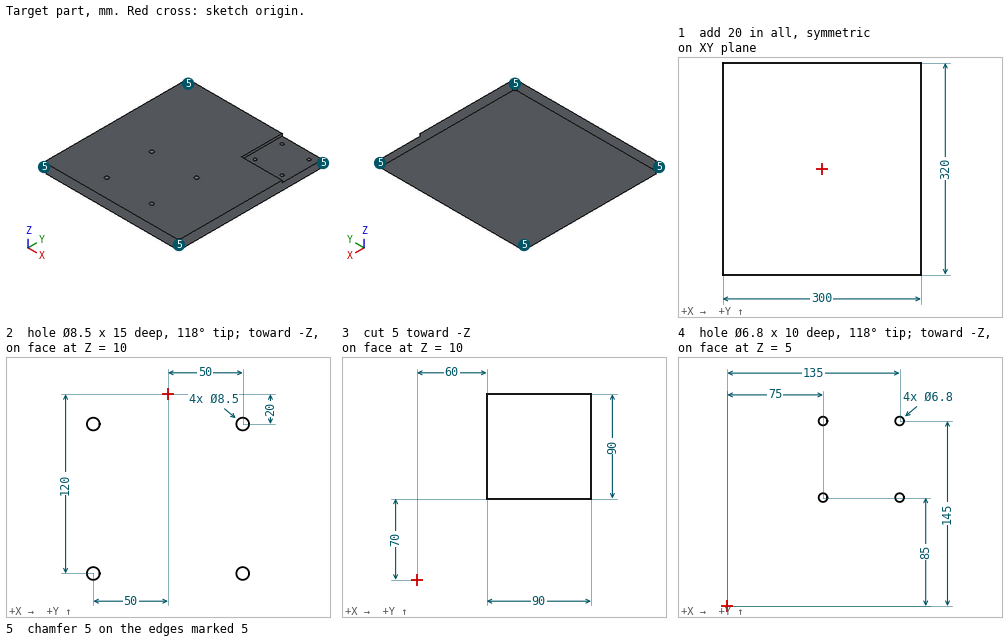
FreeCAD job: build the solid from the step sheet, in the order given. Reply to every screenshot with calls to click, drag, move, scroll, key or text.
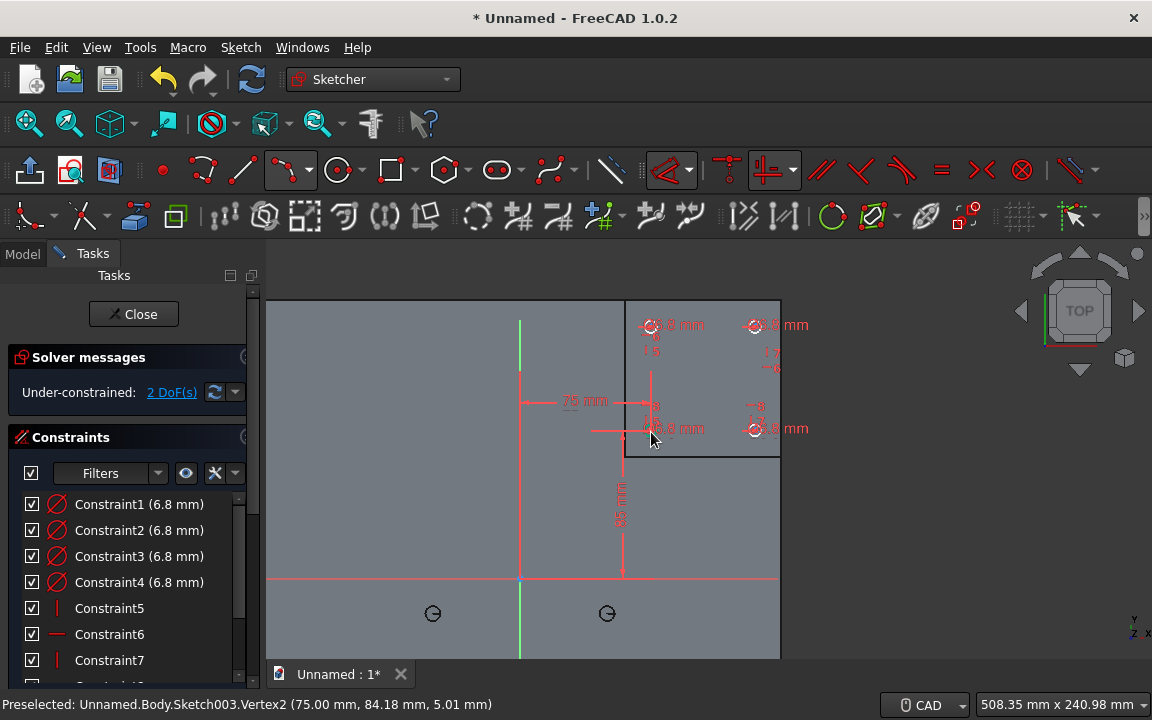
click(755, 327)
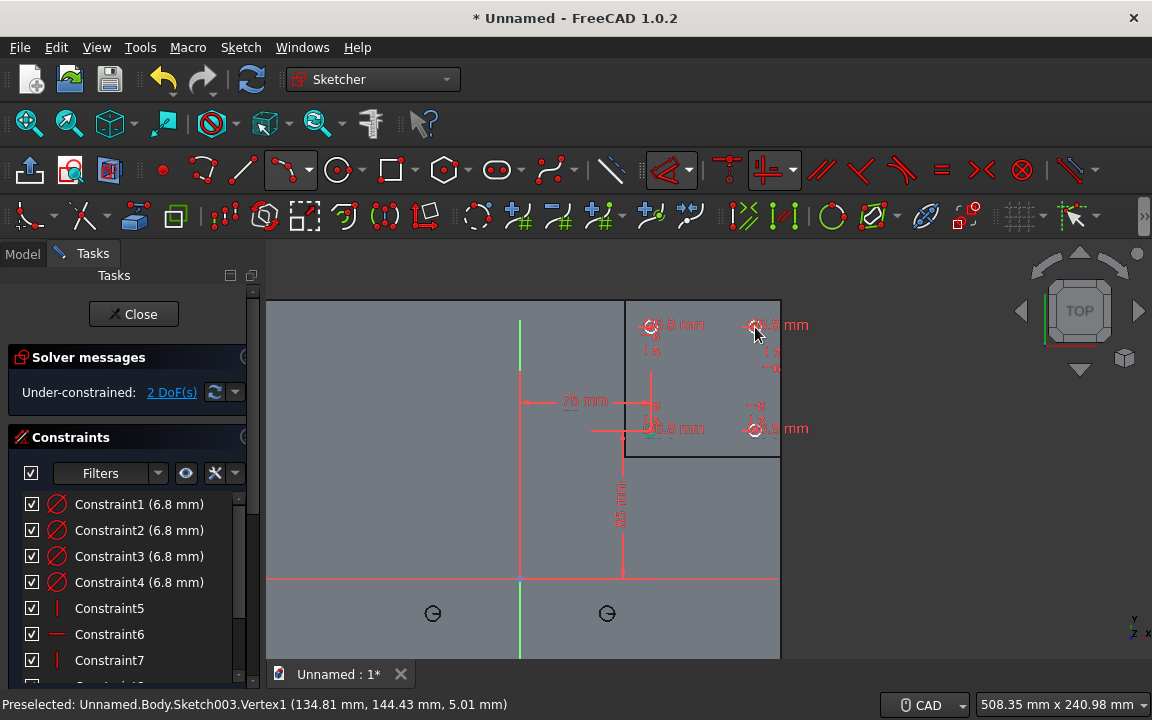
key(l)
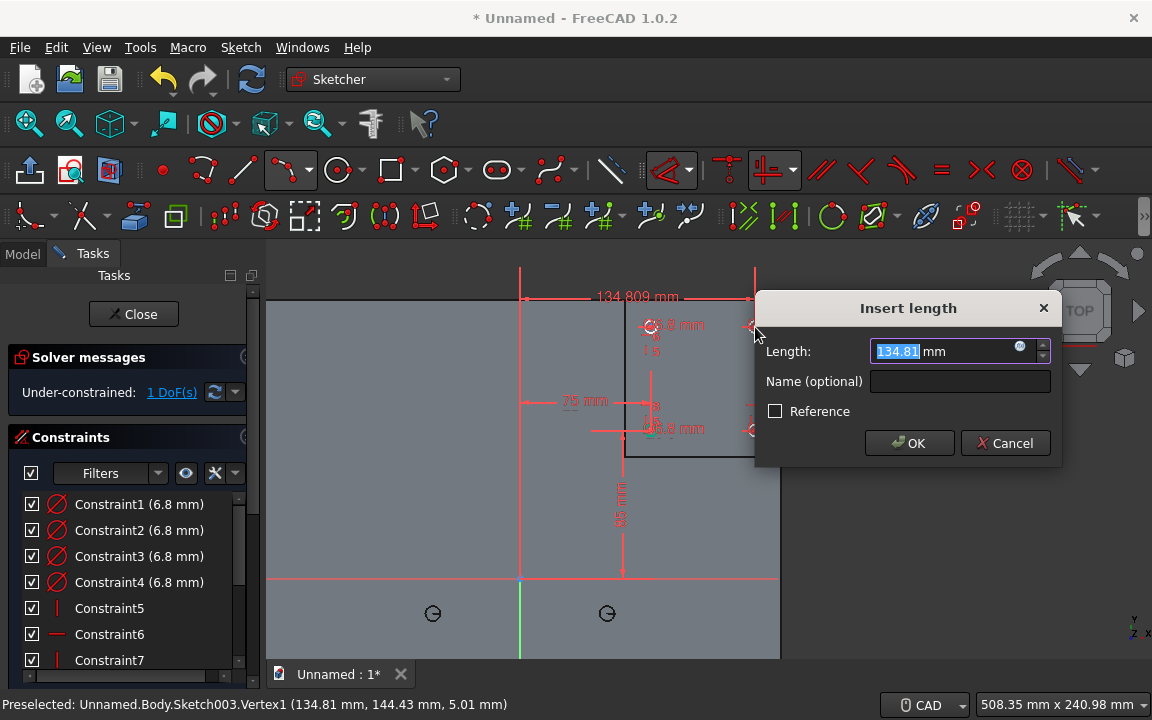
text(135)
key(Return)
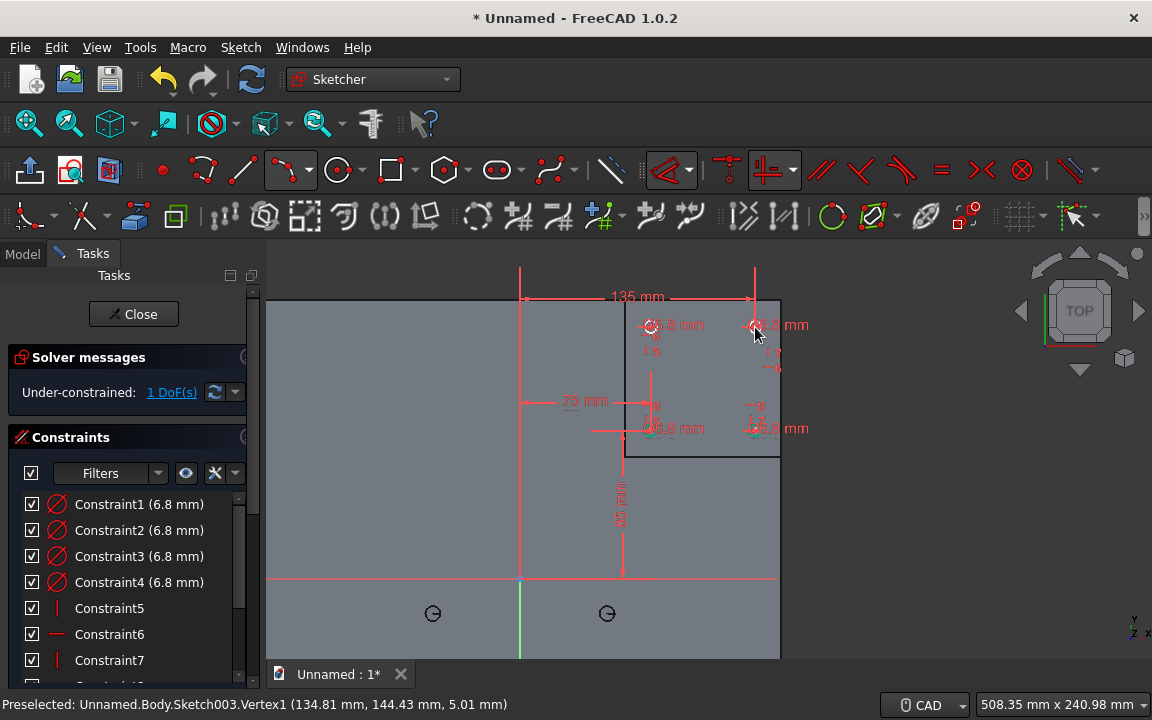
click(755, 327)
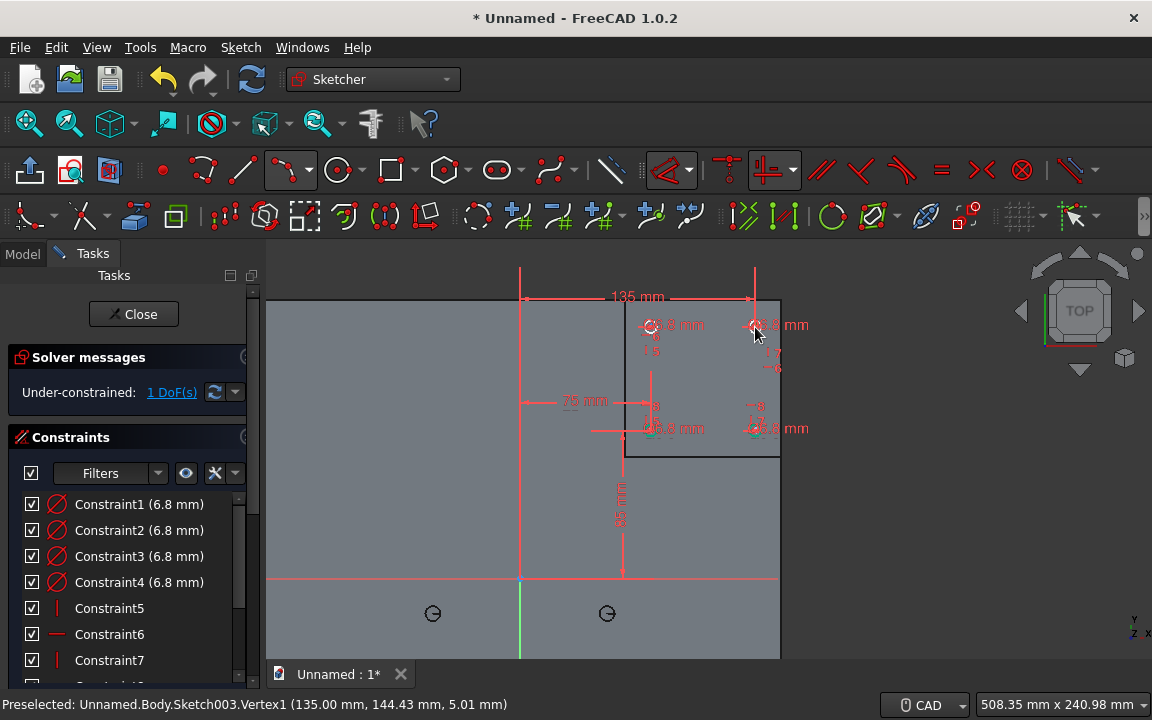
key(i)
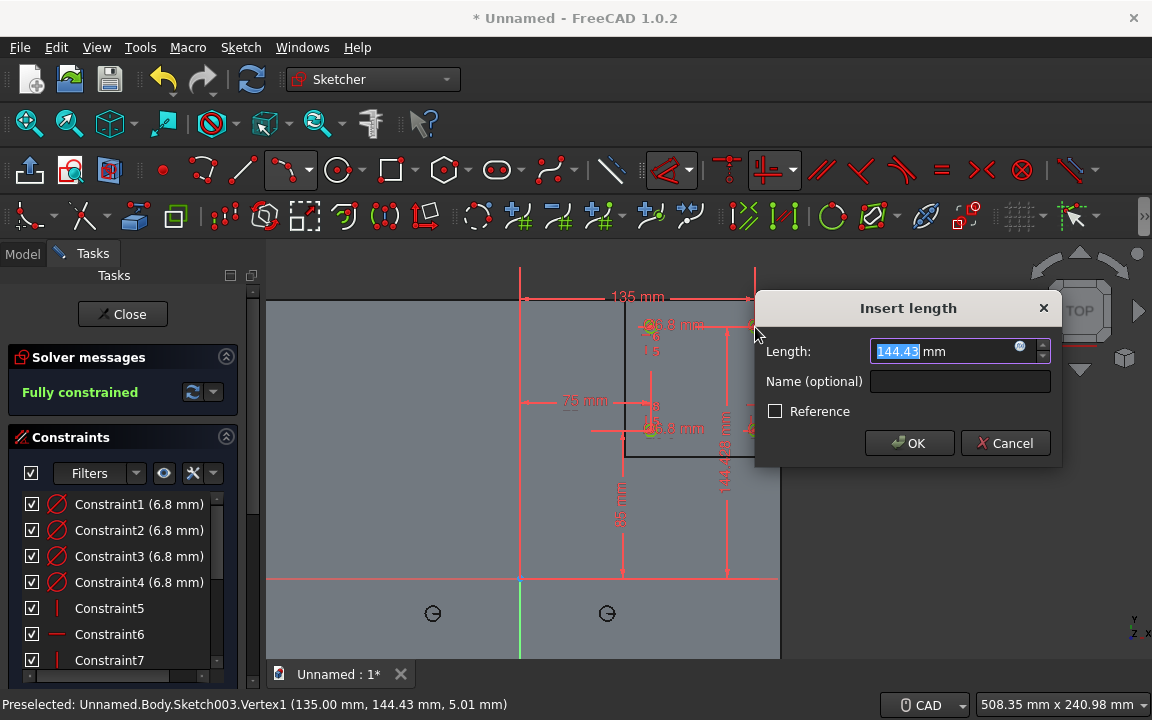
text(145)
key(Return)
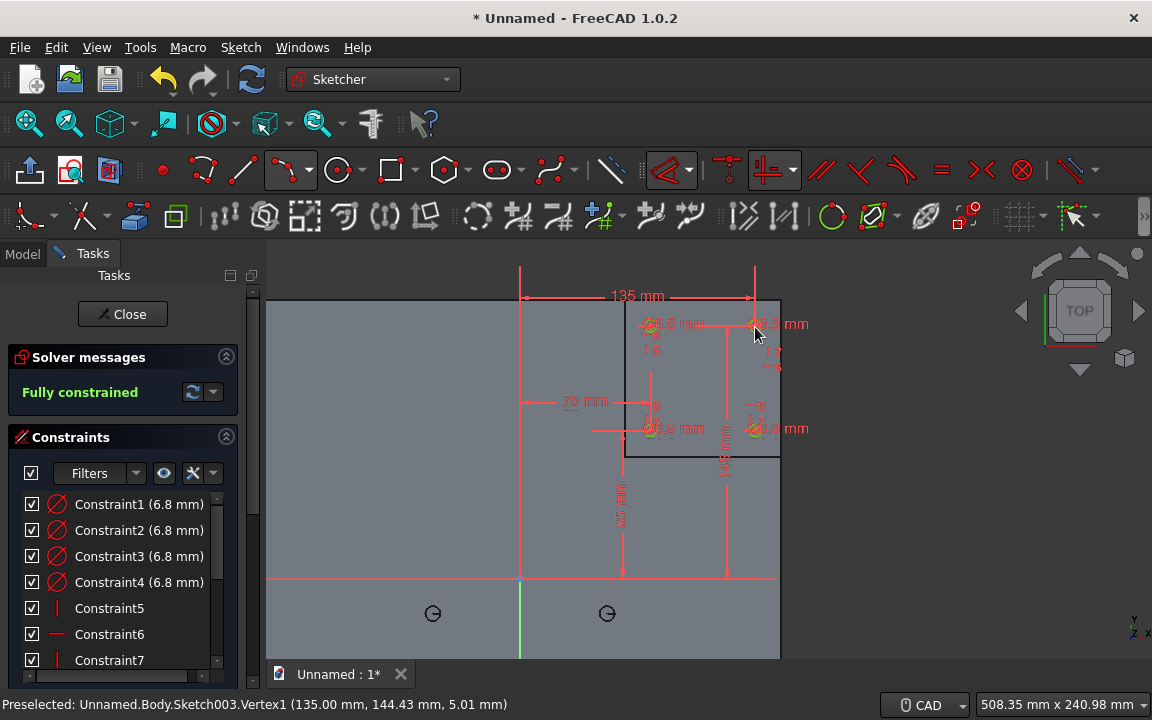
click(123, 314)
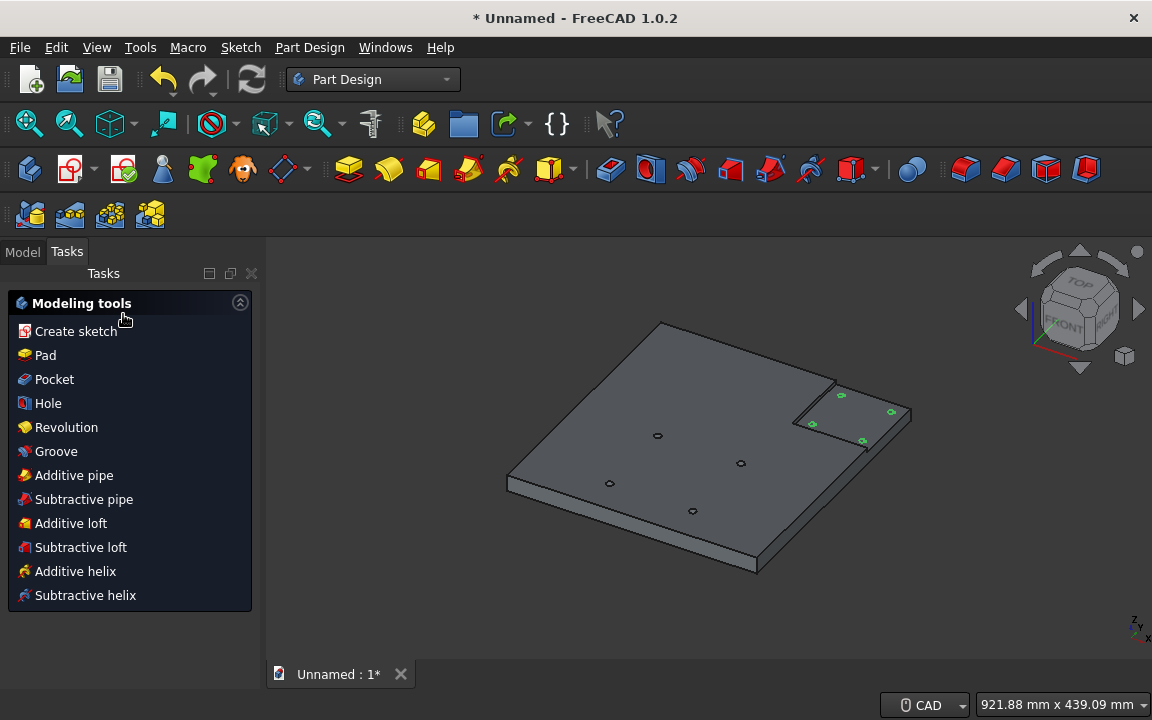
click(652, 170)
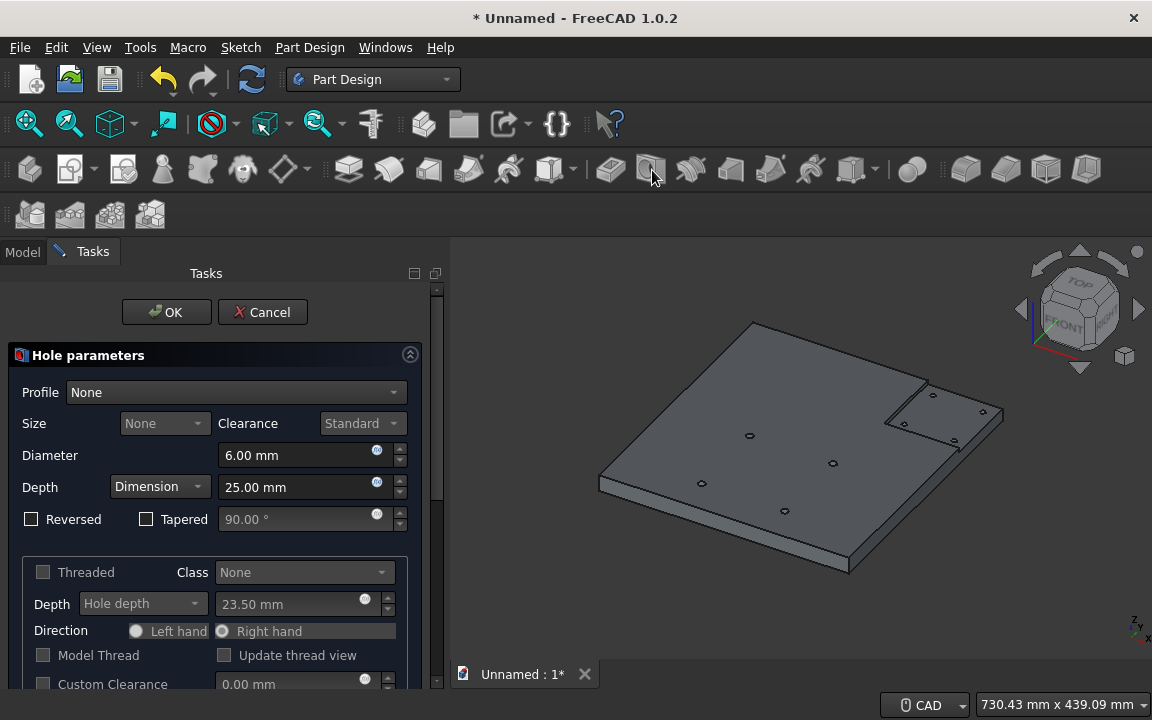
triple_click(305, 455)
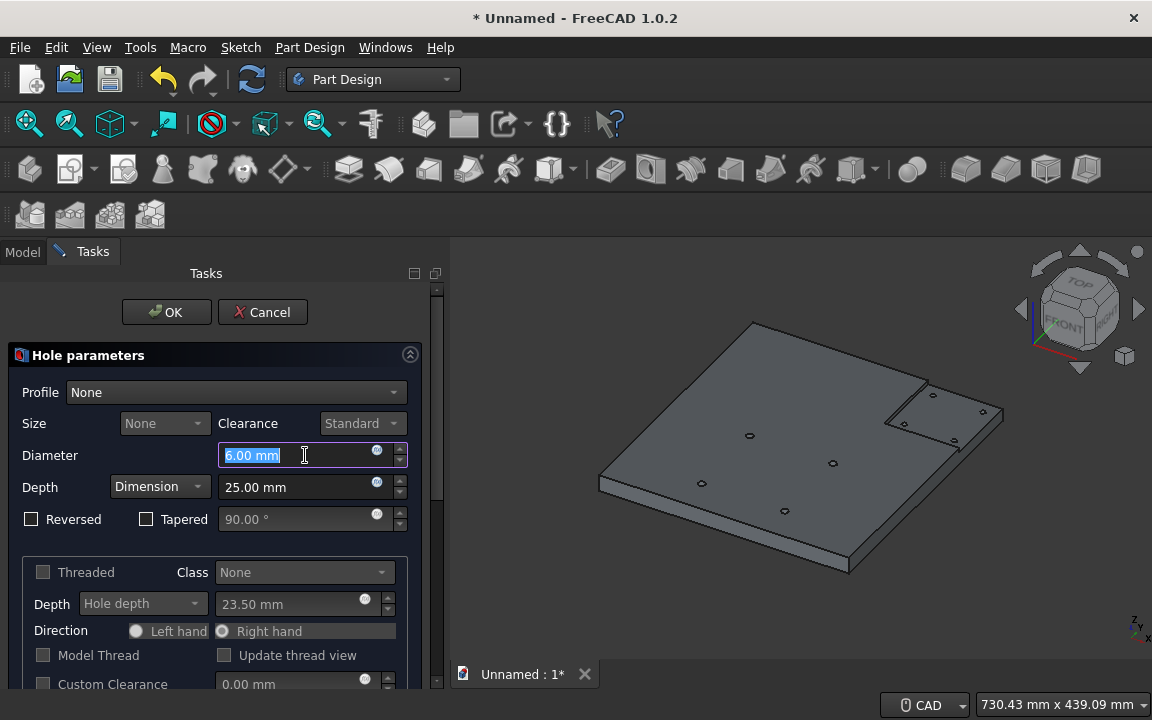
text(6.8)
key(Tab)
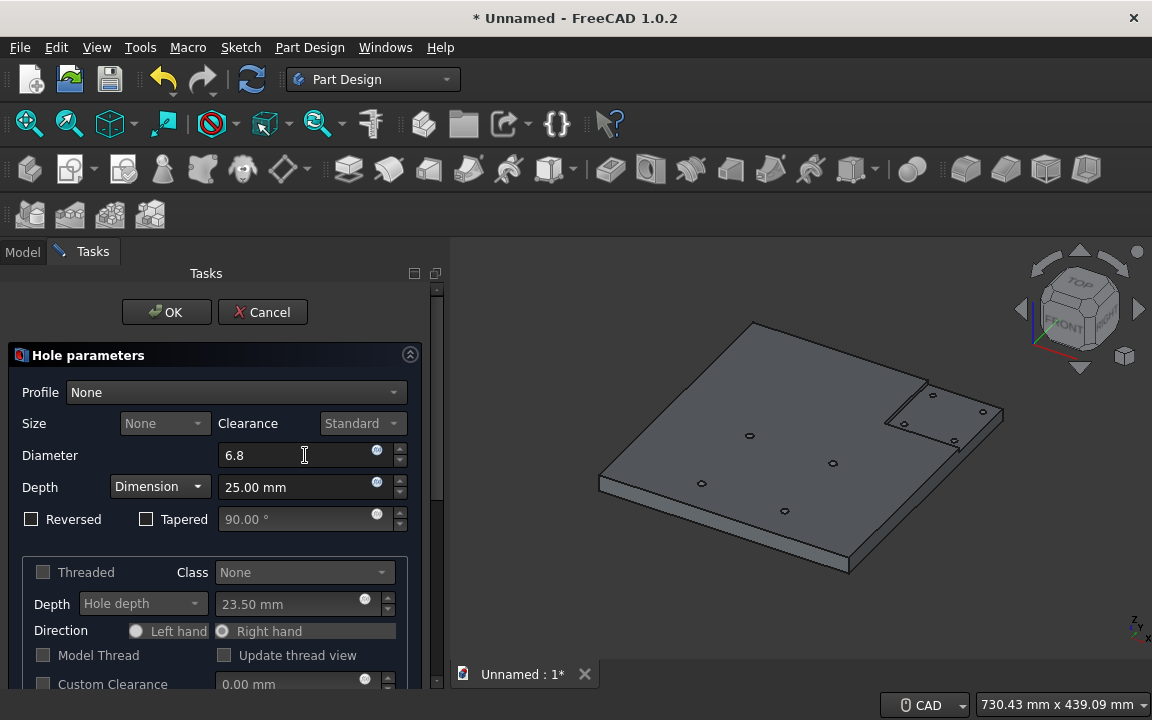
triple_click(305, 487)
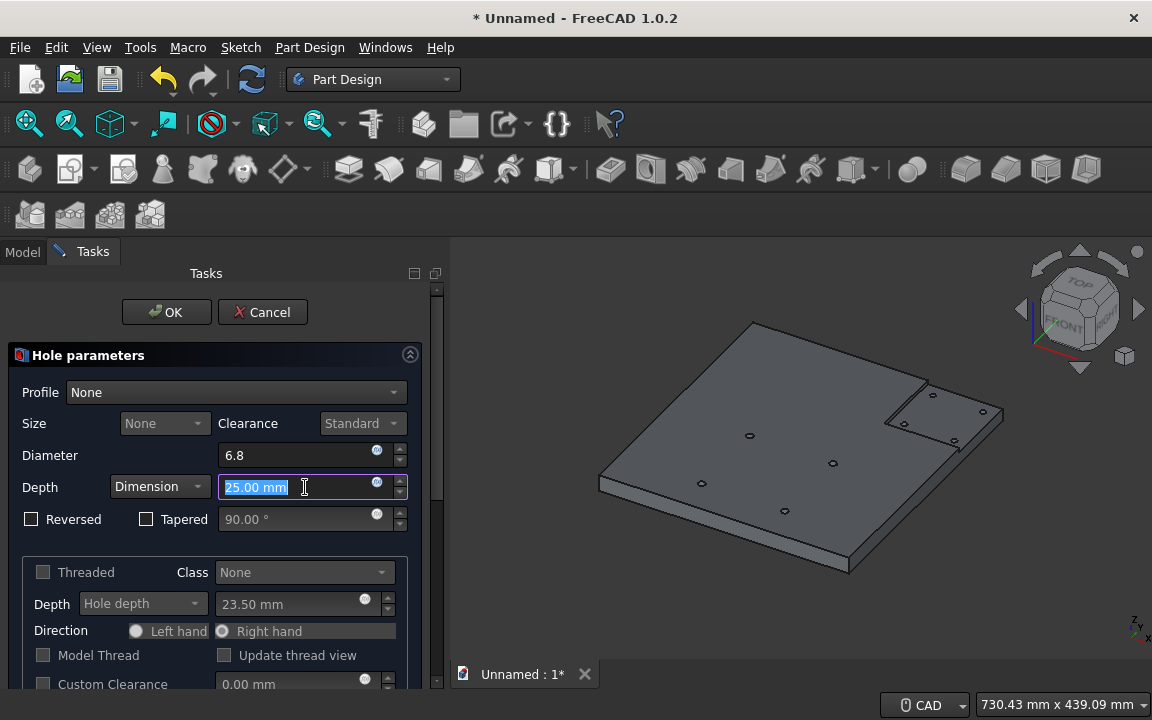
text(10)
key(Tab)